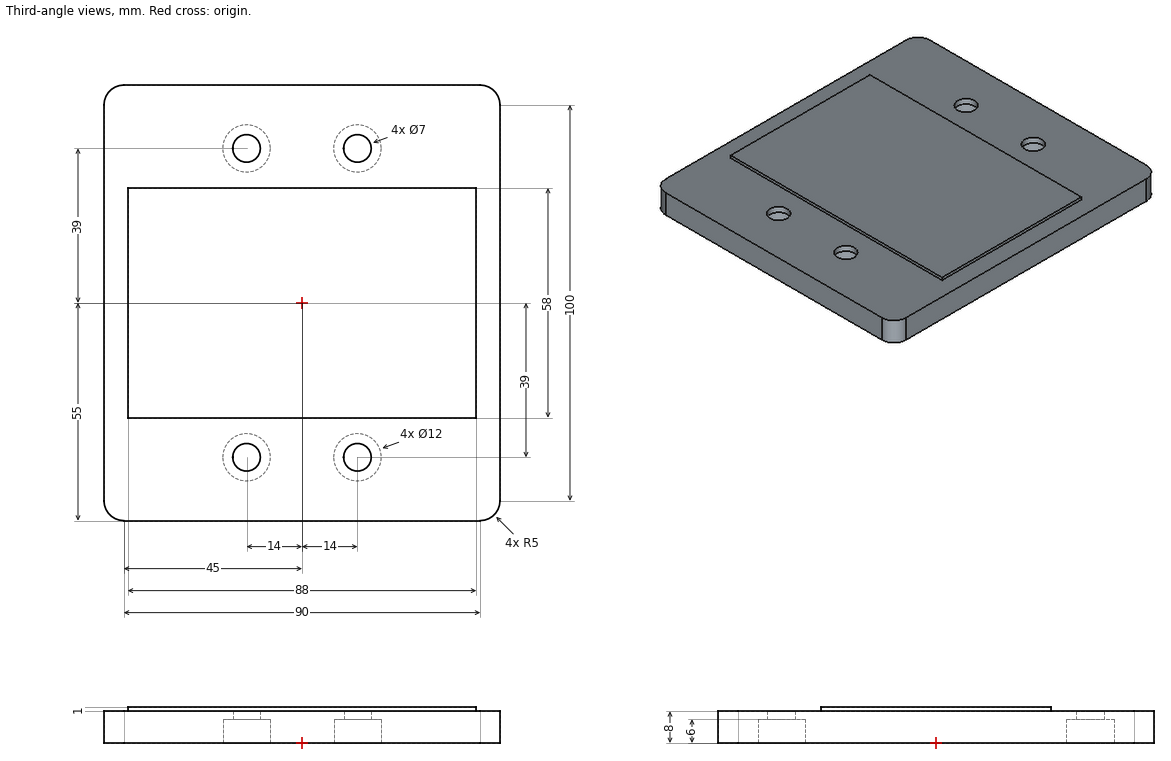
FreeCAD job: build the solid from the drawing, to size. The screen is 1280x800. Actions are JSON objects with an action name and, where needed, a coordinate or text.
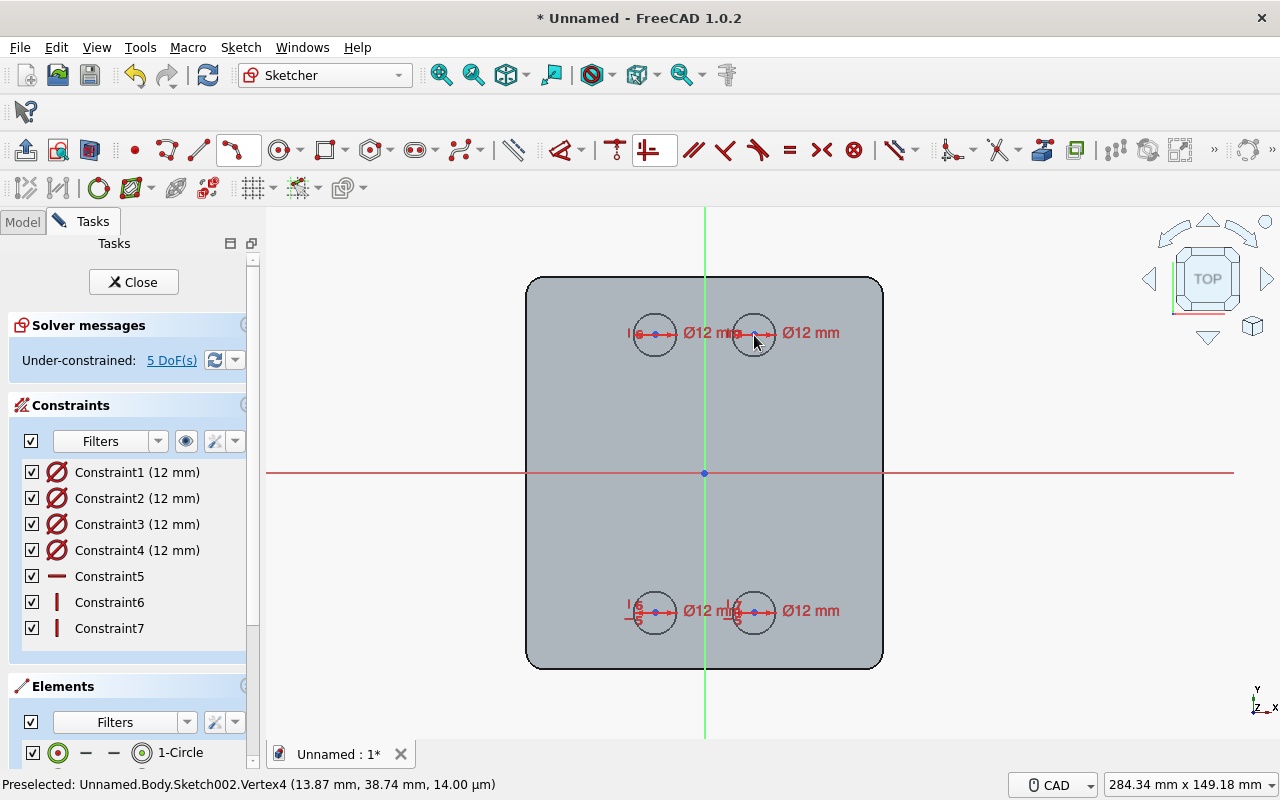
{"action": "left_click", "coordinate": [655, 335]}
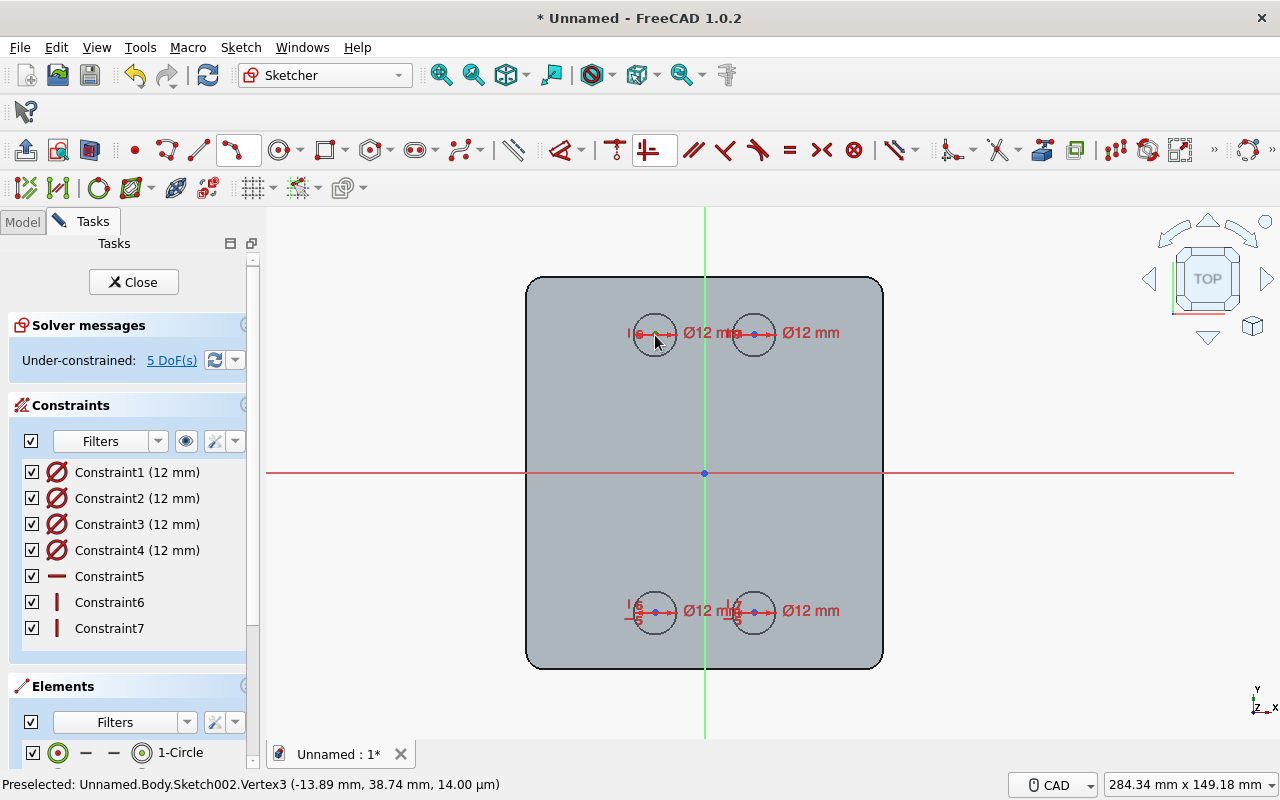
{"action": "left_click", "coordinate": [754, 335]}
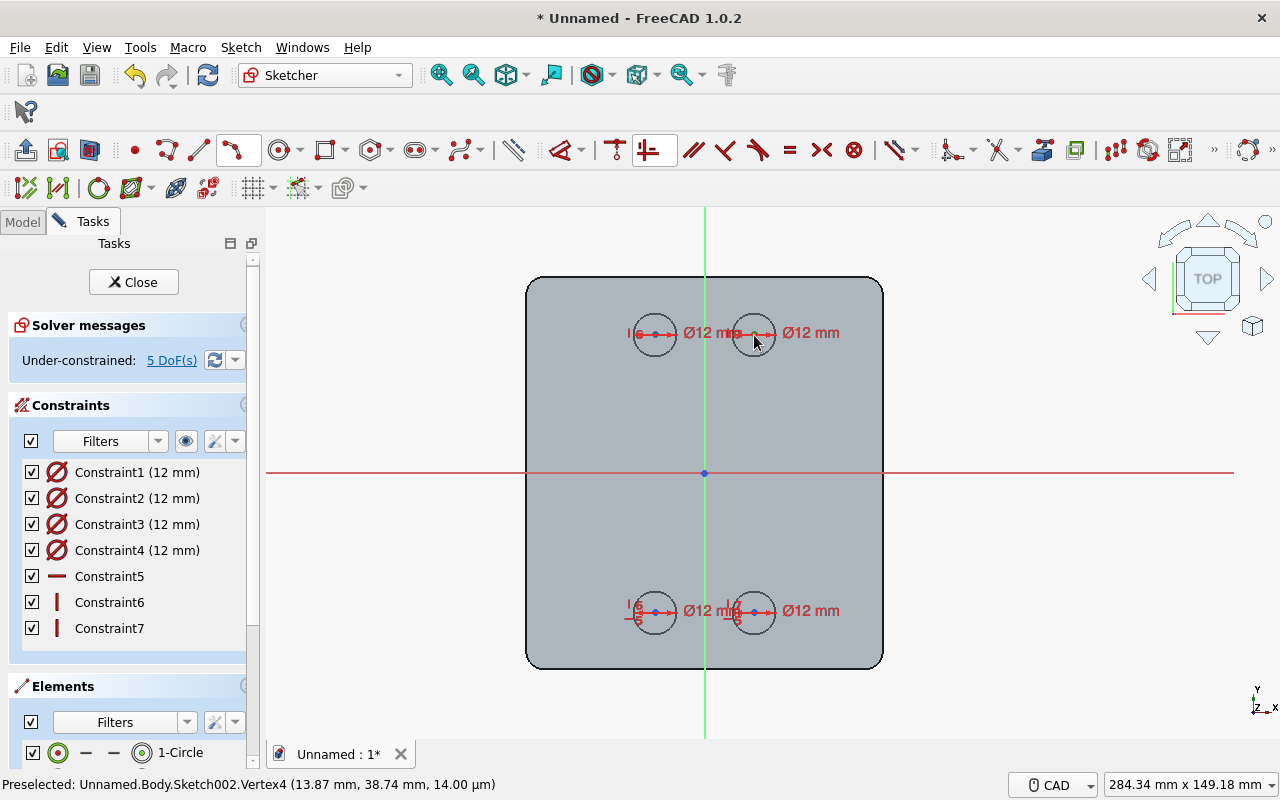
{"action": "key", "text": "h"}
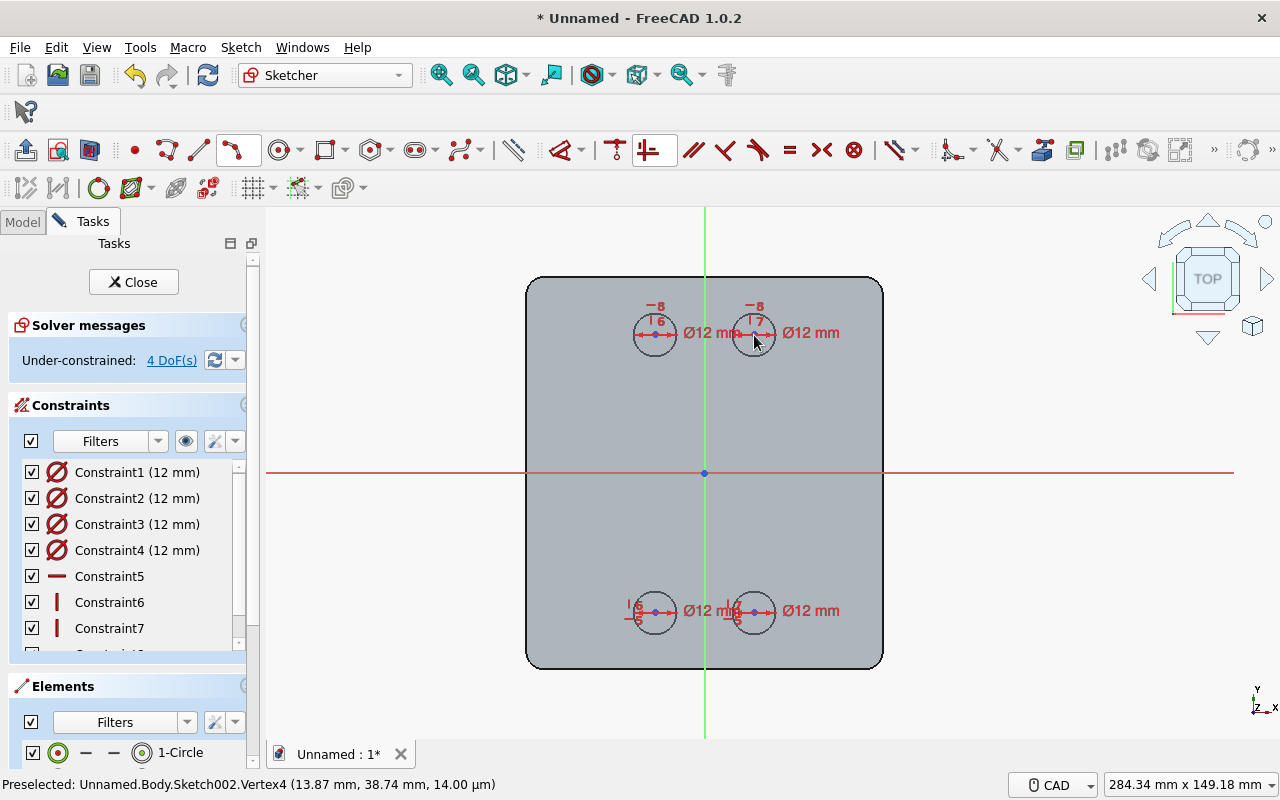
{"action": "left_click", "coordinate": [560, 150]}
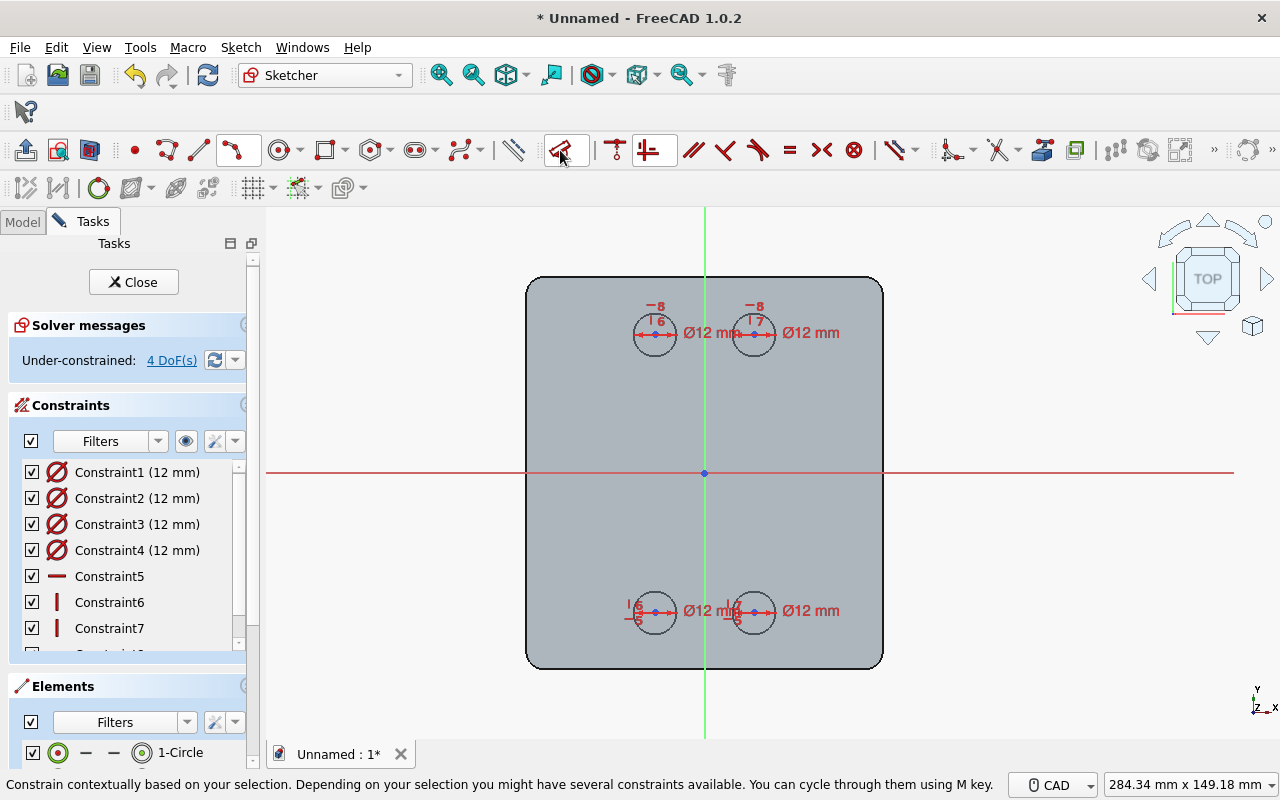
{"action": "left_click", "coordinate": [754, 613]}
{"action": "left_click", "coordinate": [729, 647]}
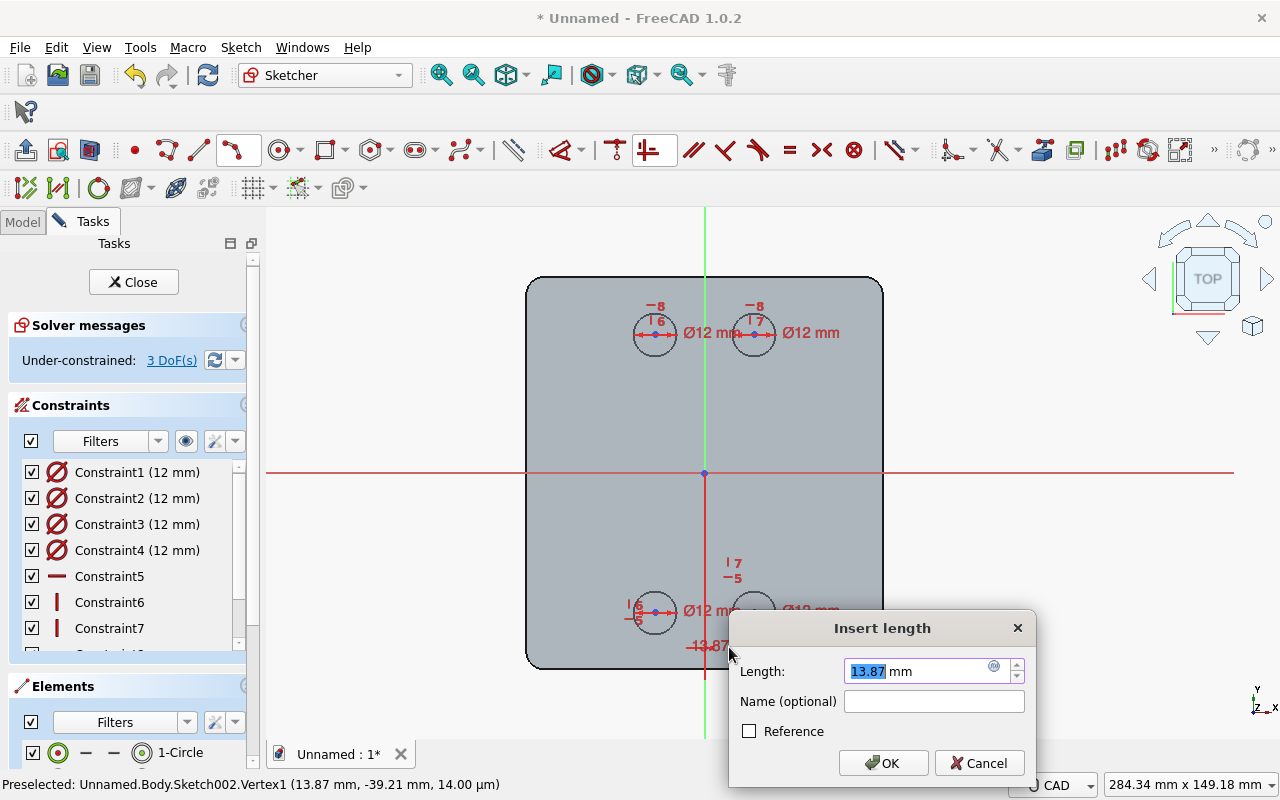
{"action": "type", "text": "14"}
{"action": "key", "text": "Return"}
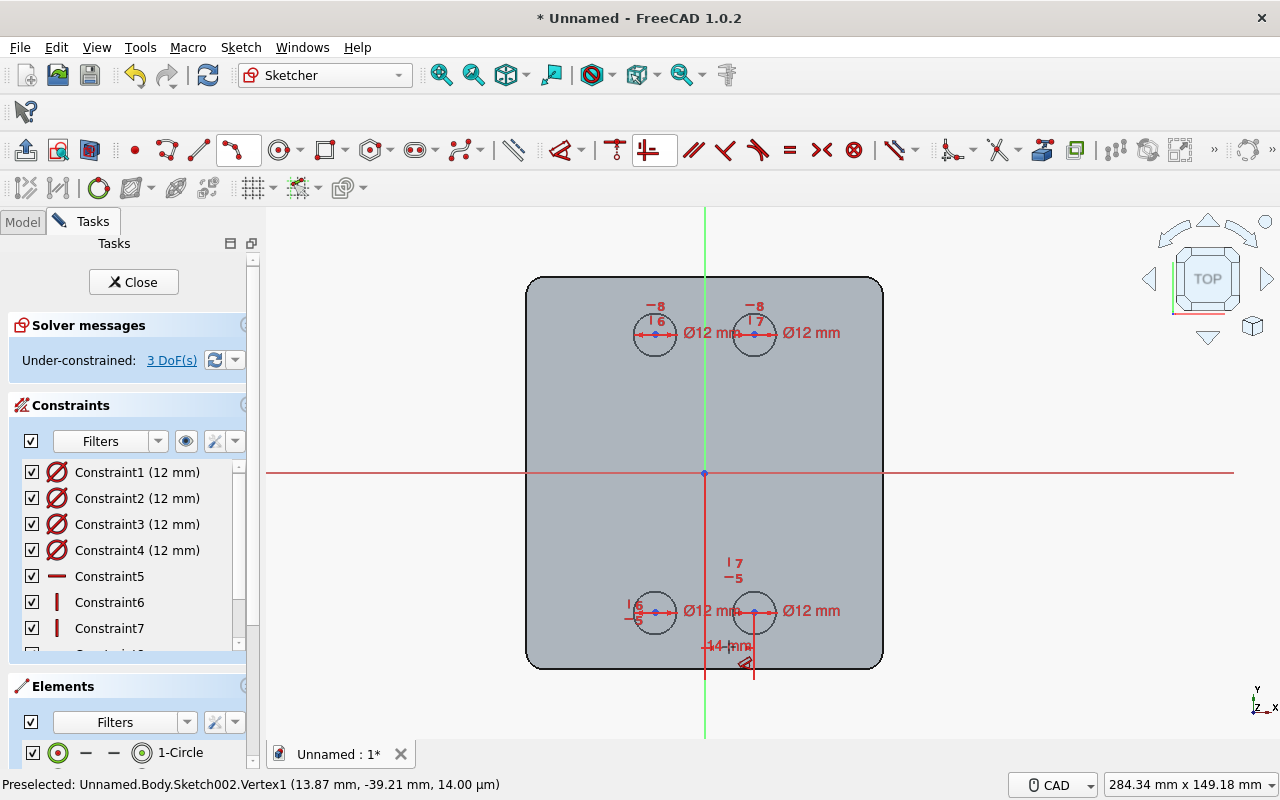
{"action": "left_click", "coordinate": [754, 613]}
{"action": "left_click", "coordinate": [788, 543]}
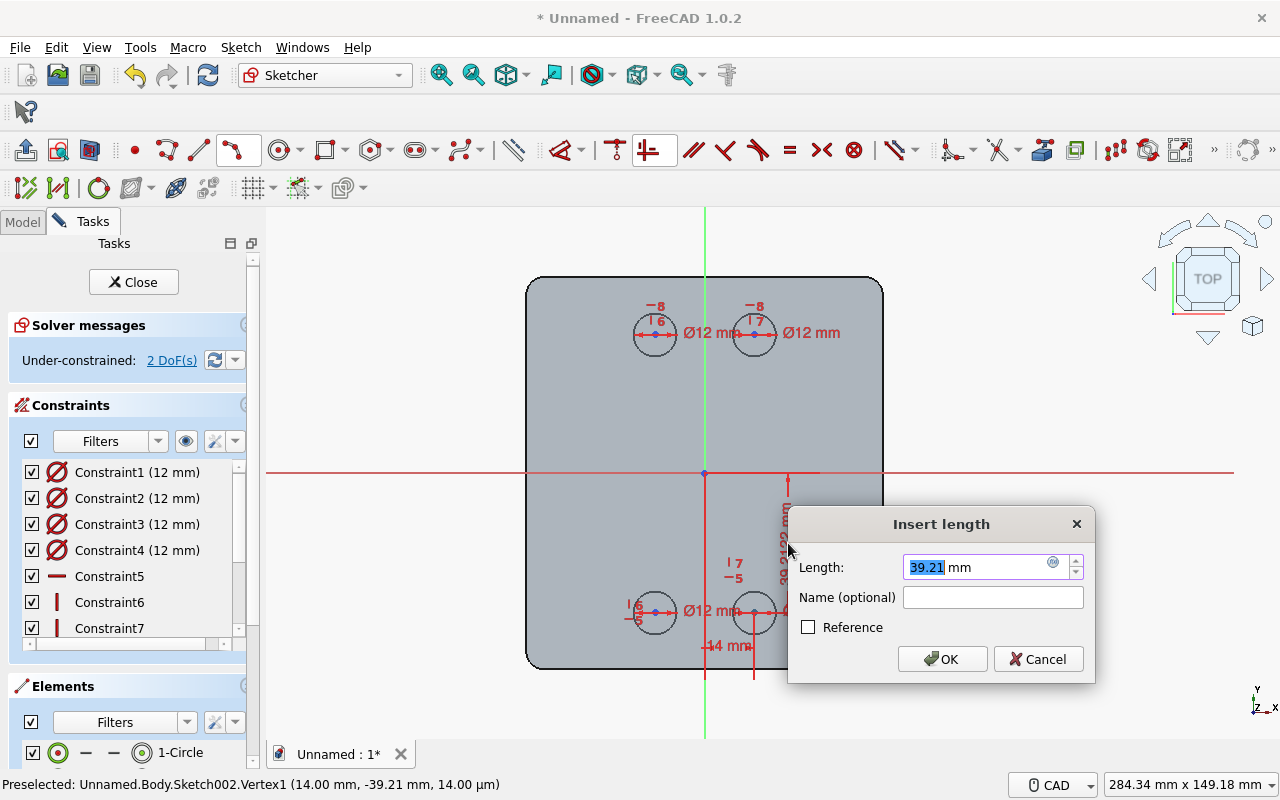
{"action": "type", "text": "39"}
{"action": "key", "text": "Return"}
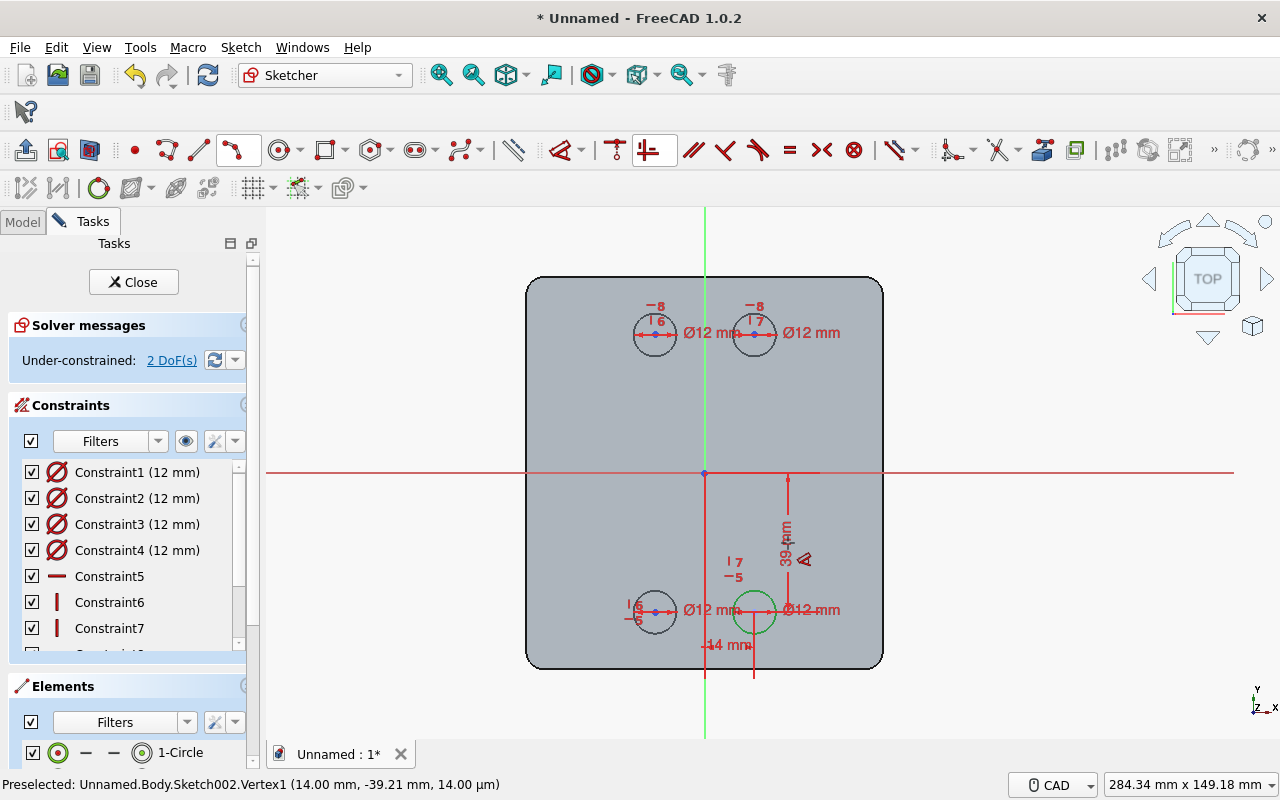
{"action": "left_click", "coordinate": [655, 612]}
{"action": "left_click", "coordinate": [680, 439]}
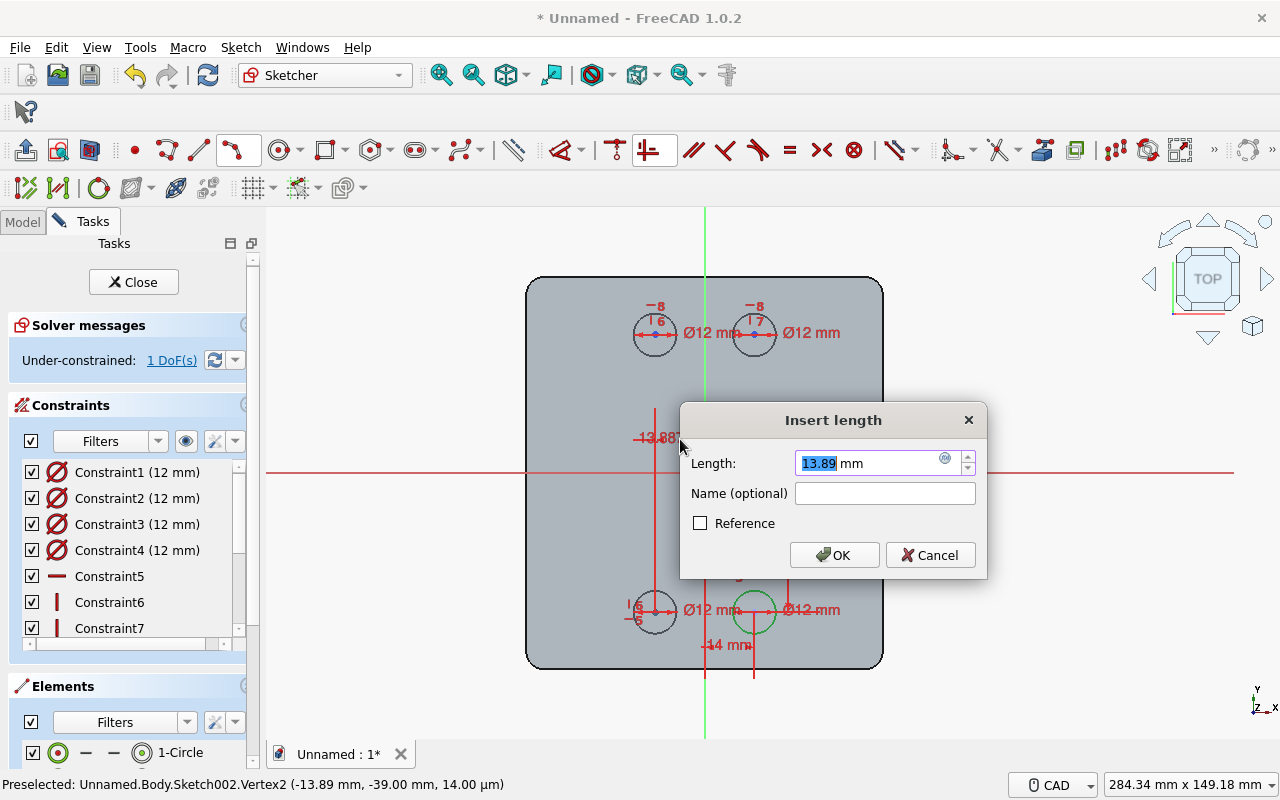
{"action": "type", "text": "14"}
{"action": "key", "text": "Return"}